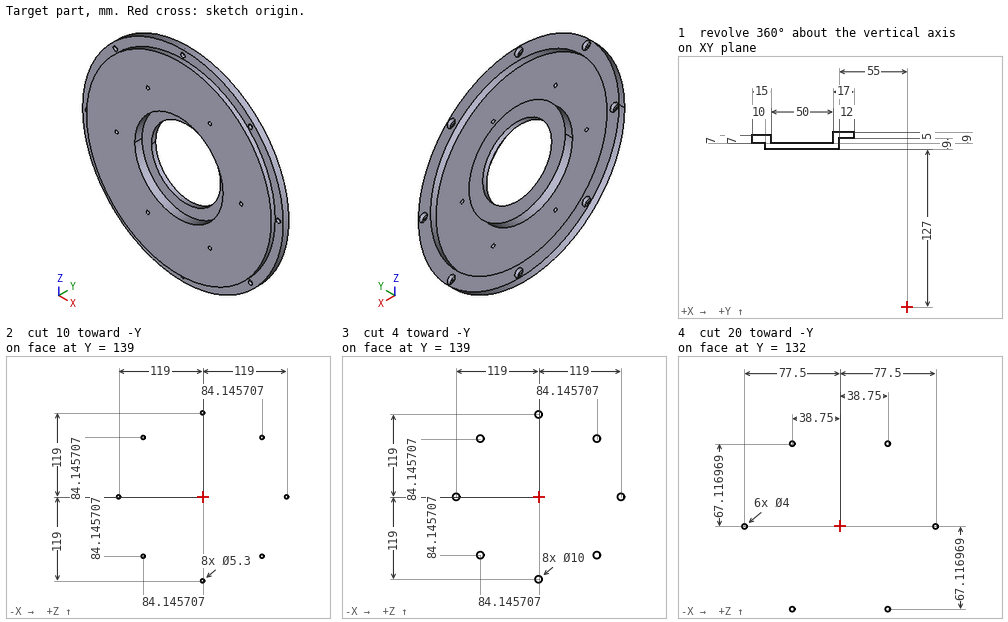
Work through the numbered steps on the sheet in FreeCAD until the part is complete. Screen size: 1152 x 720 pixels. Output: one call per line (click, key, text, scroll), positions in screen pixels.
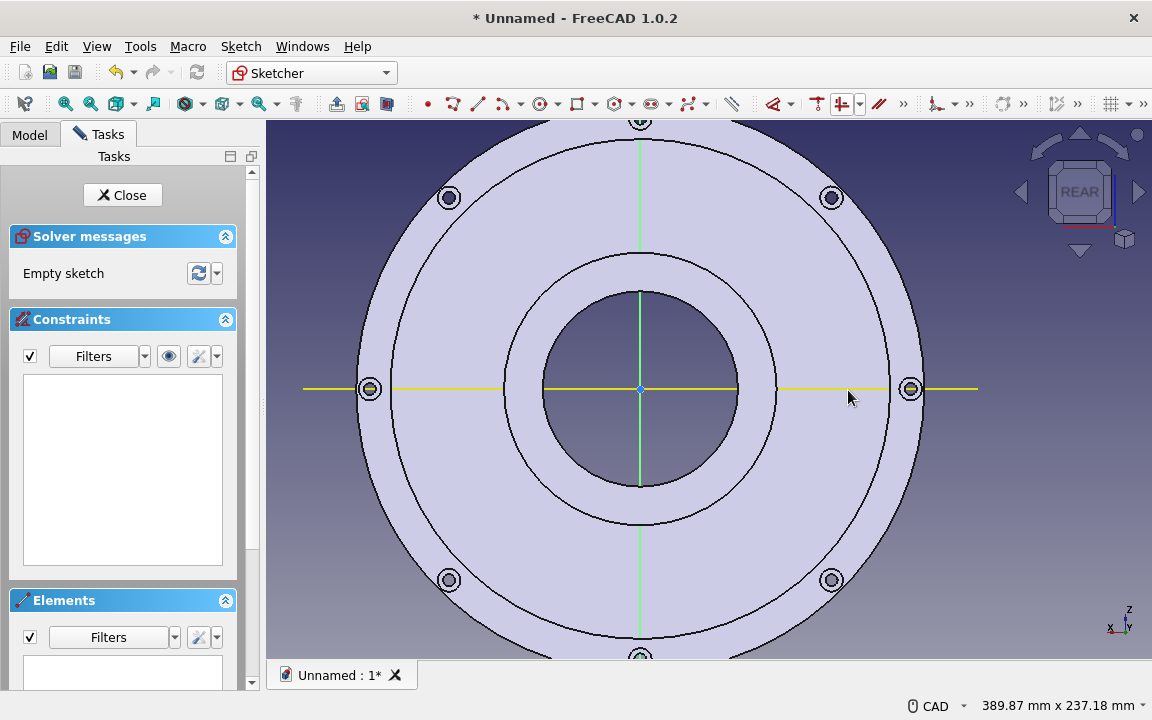
click(540, 104)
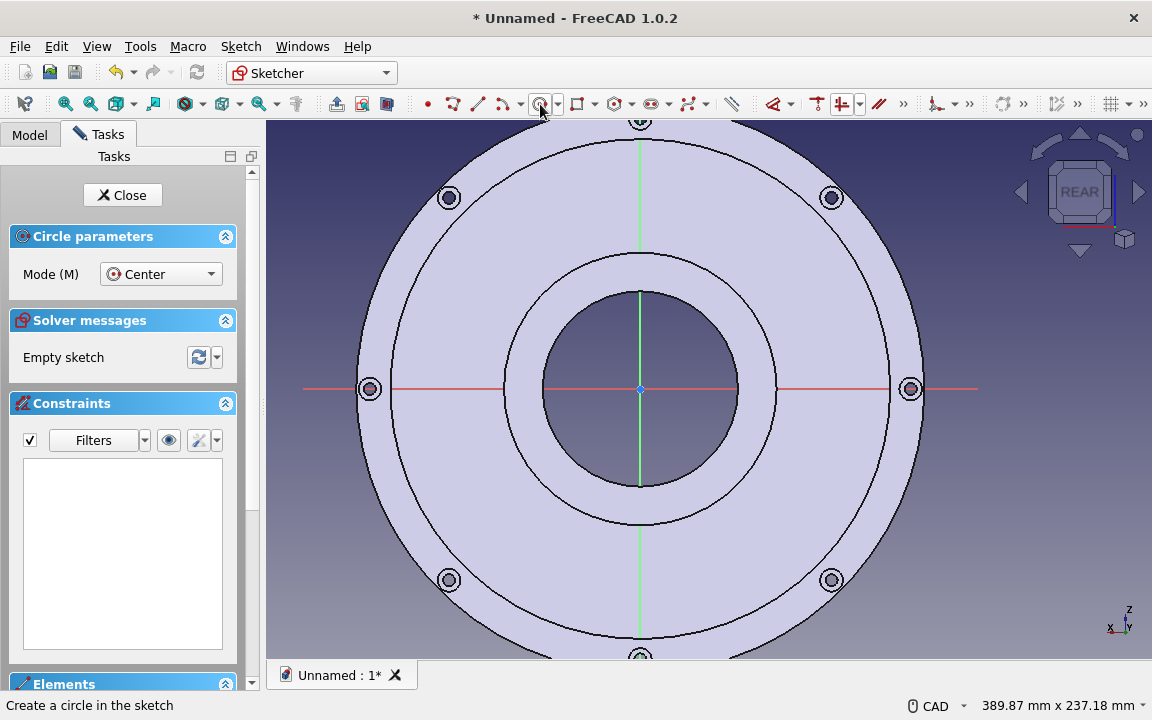
scroll(464, 389, up, 9)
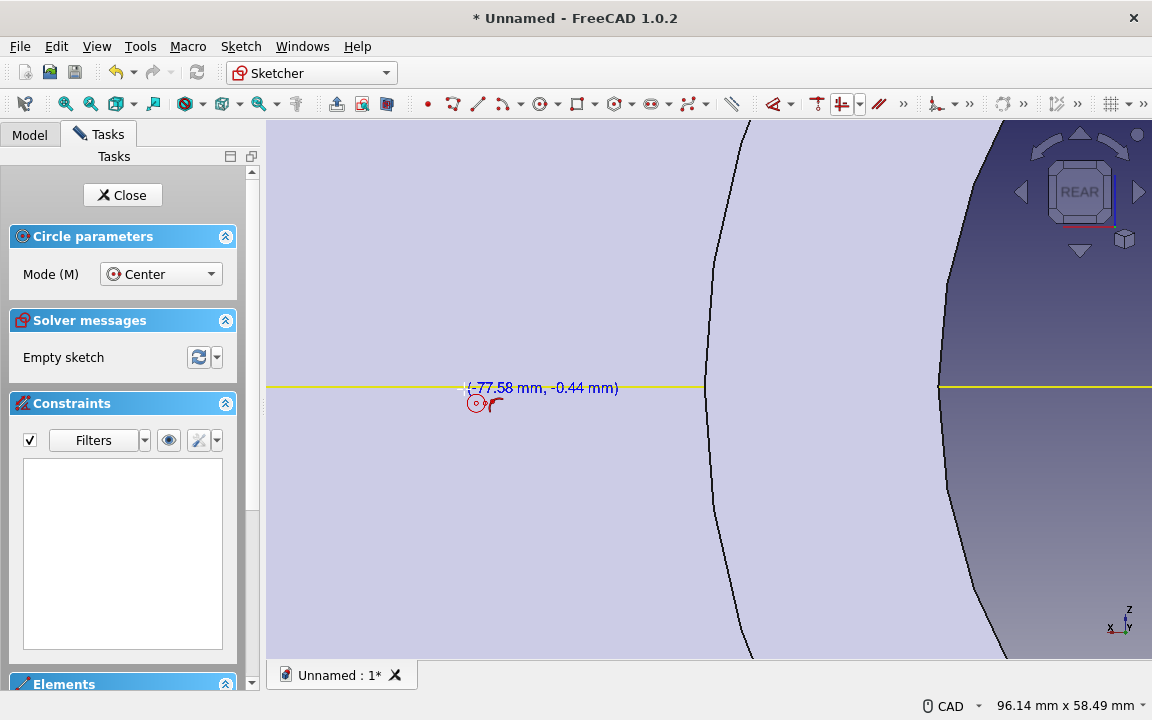
scroll(464, 390, down, 9)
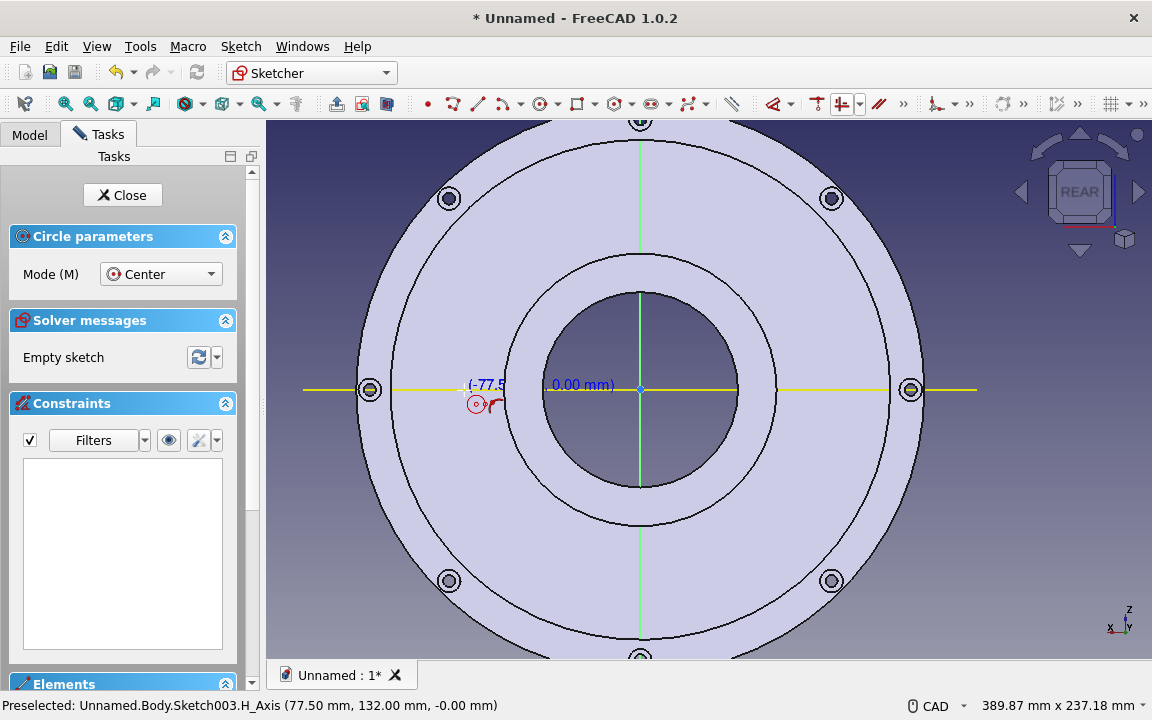
click(464, 390)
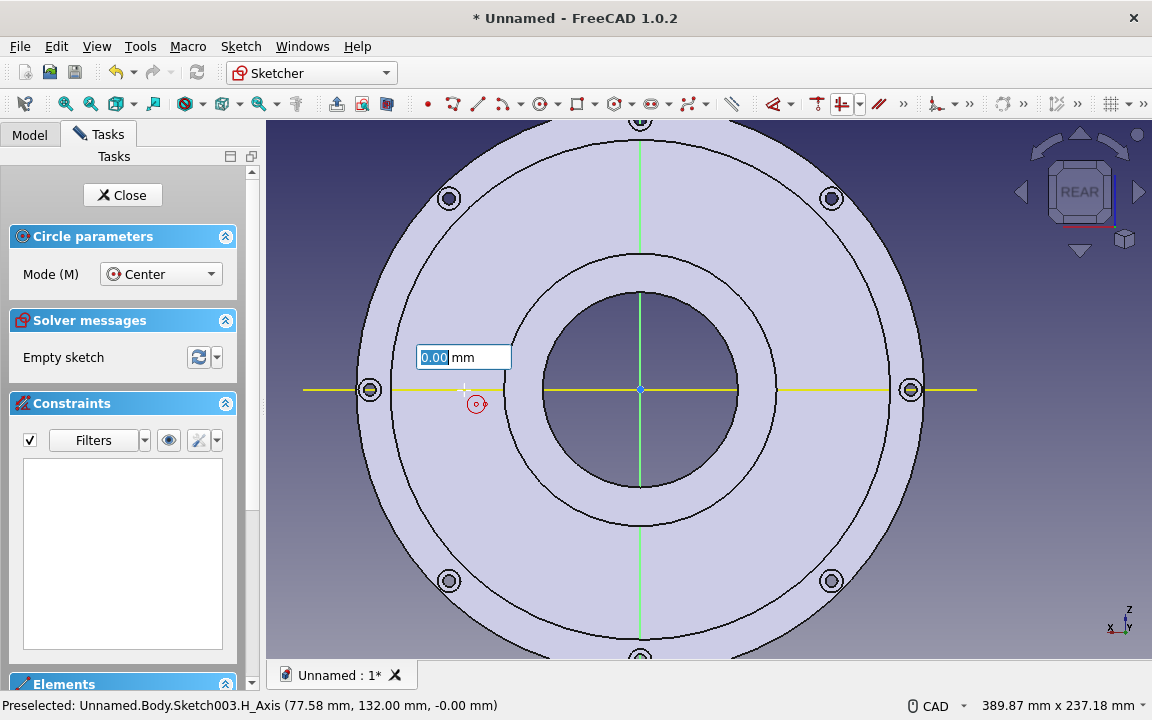
scroll(463, 394, up, 7)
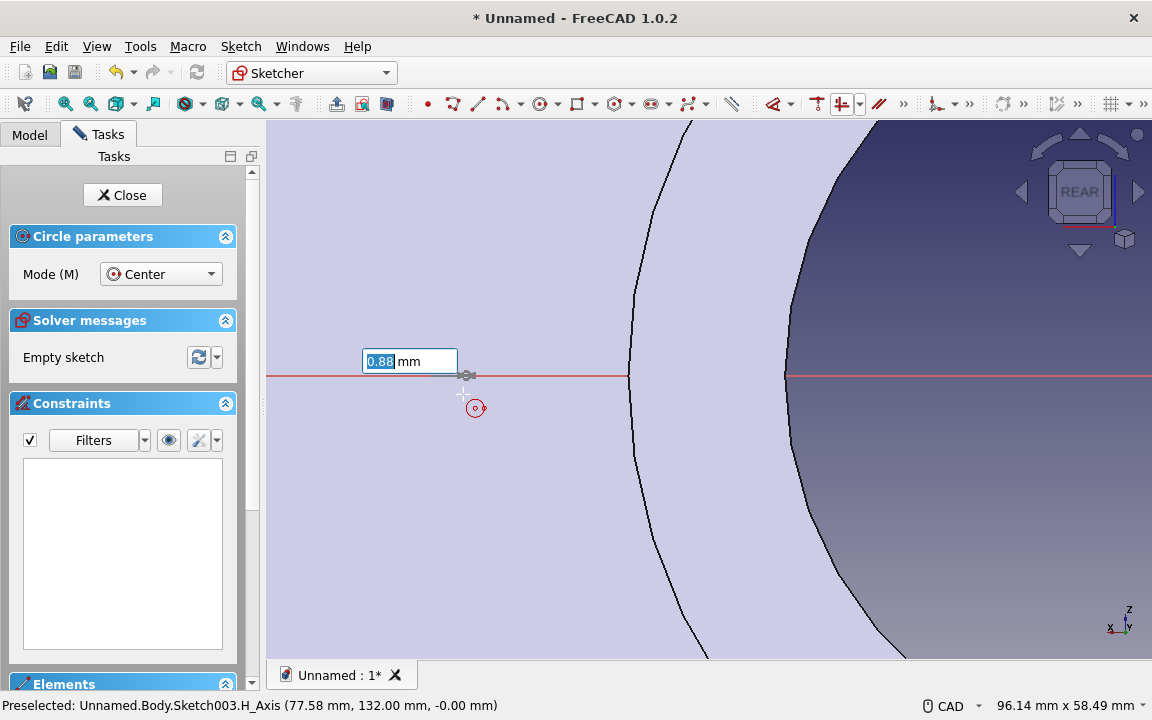
click(461, 393)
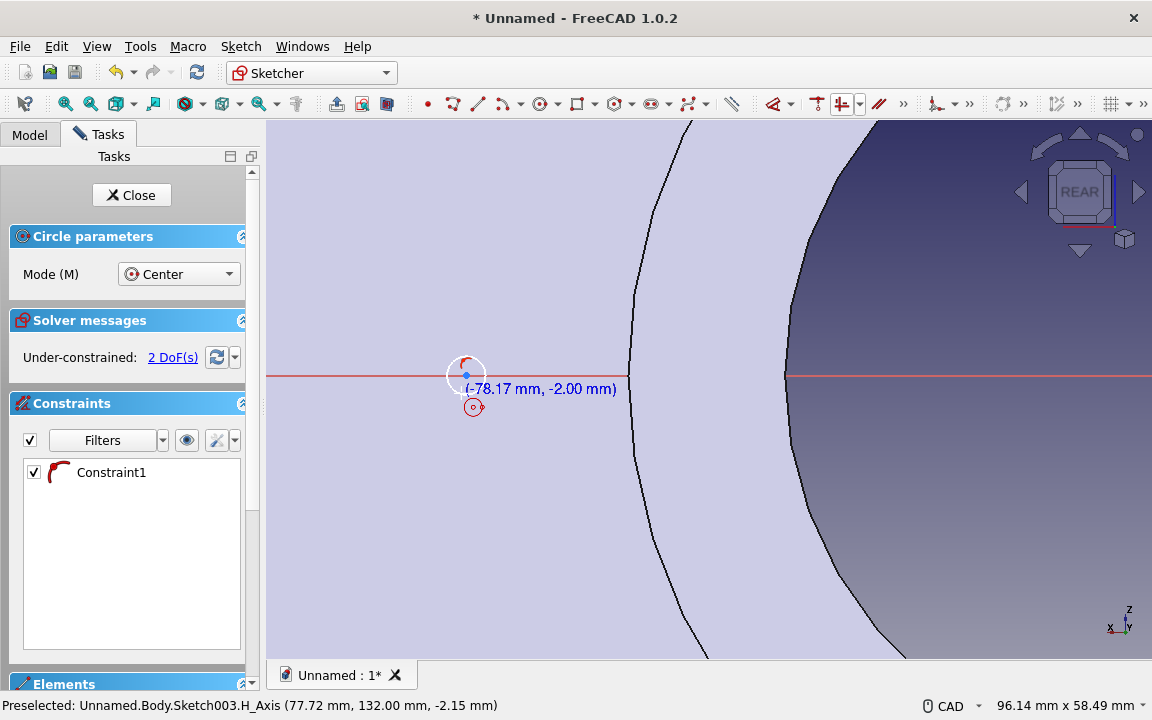
scroll(463, 394, down, 7)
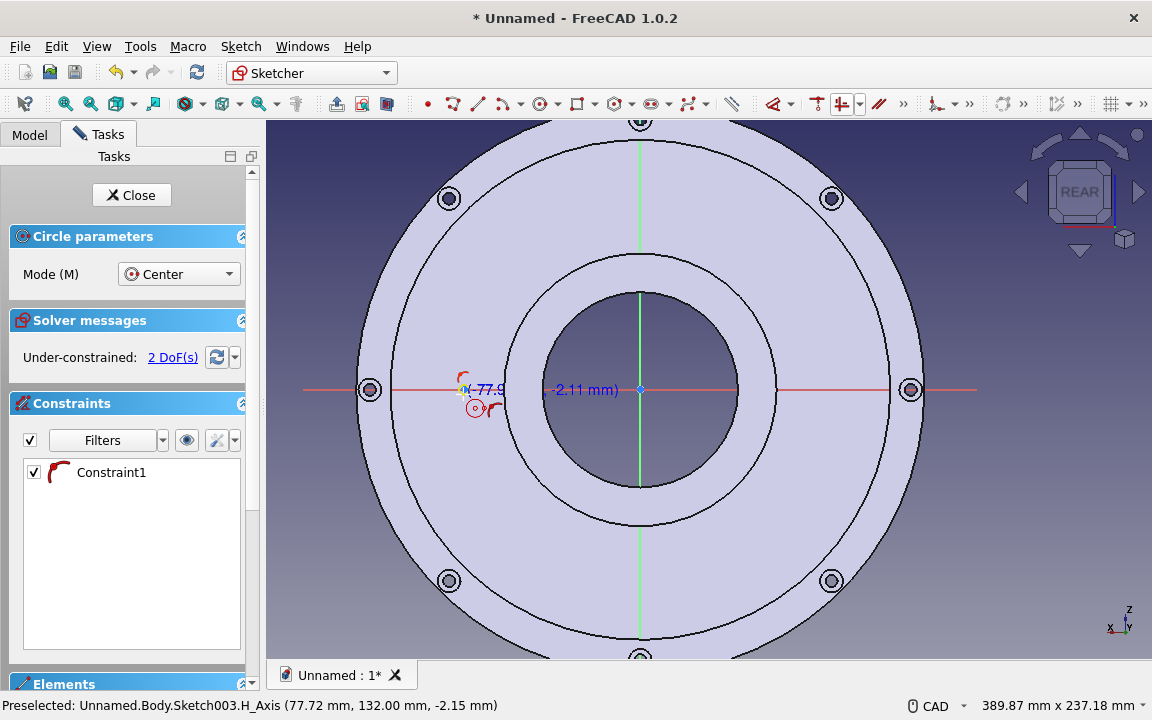
scroll(552, 237, up, 9)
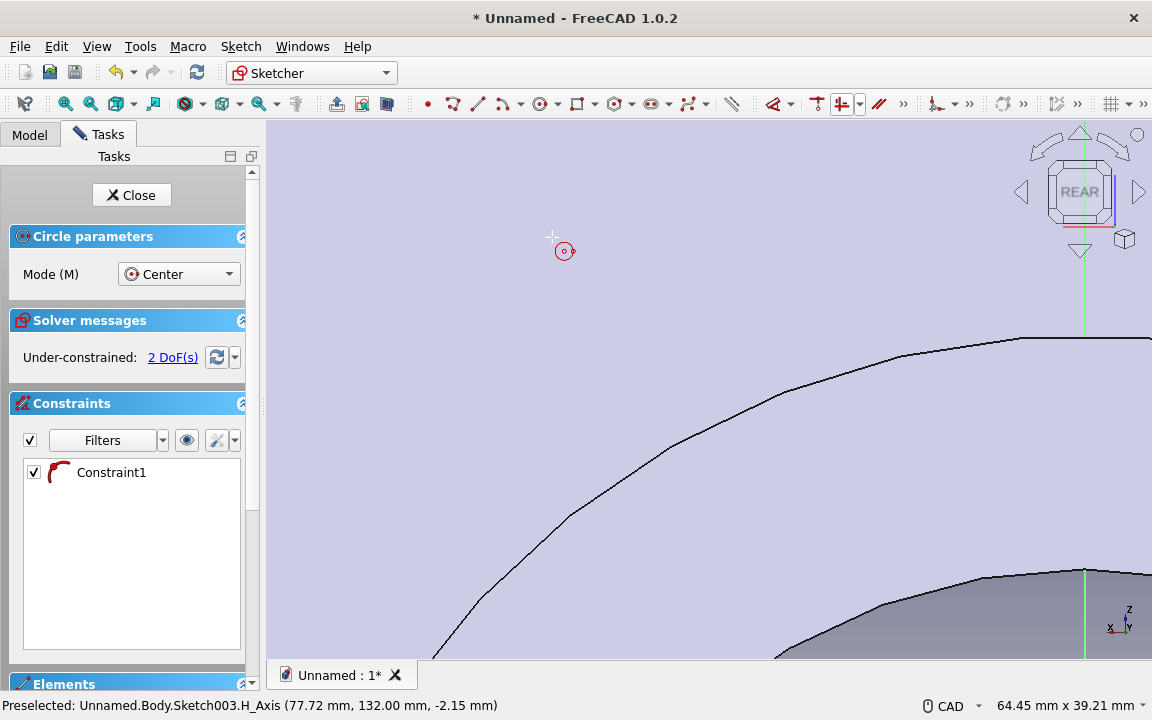
scroll(553, 237, down, 9)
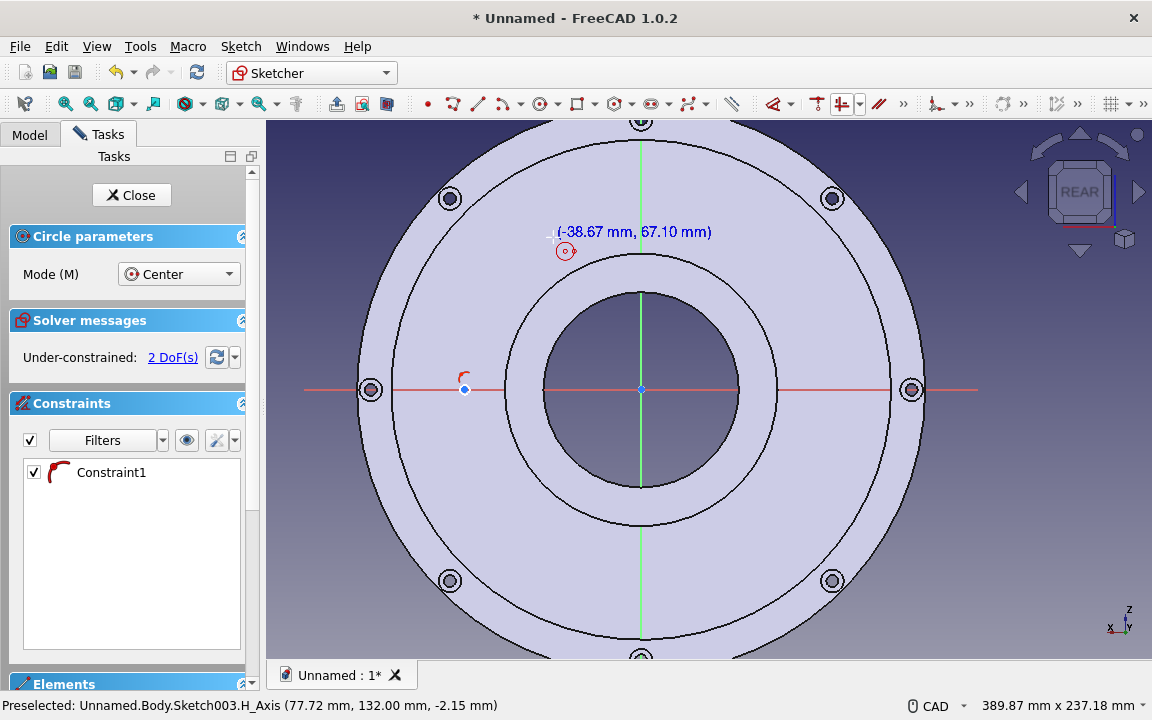
click(553, 237)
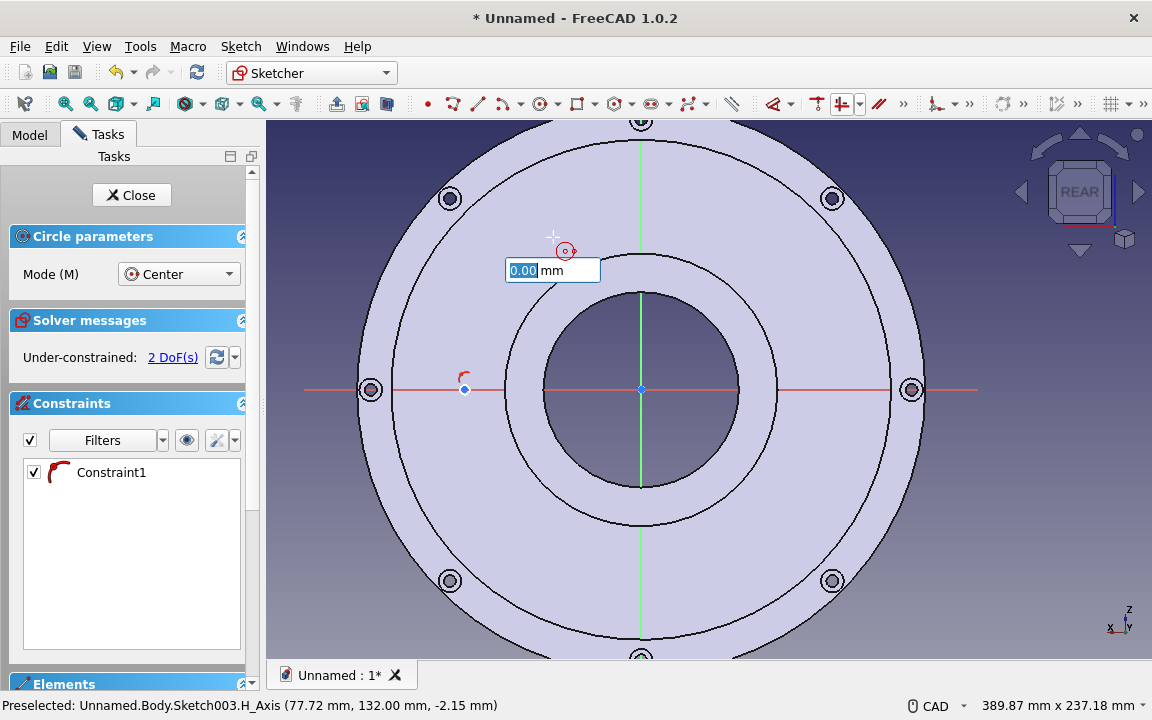
scroll(556, 234, up, 7)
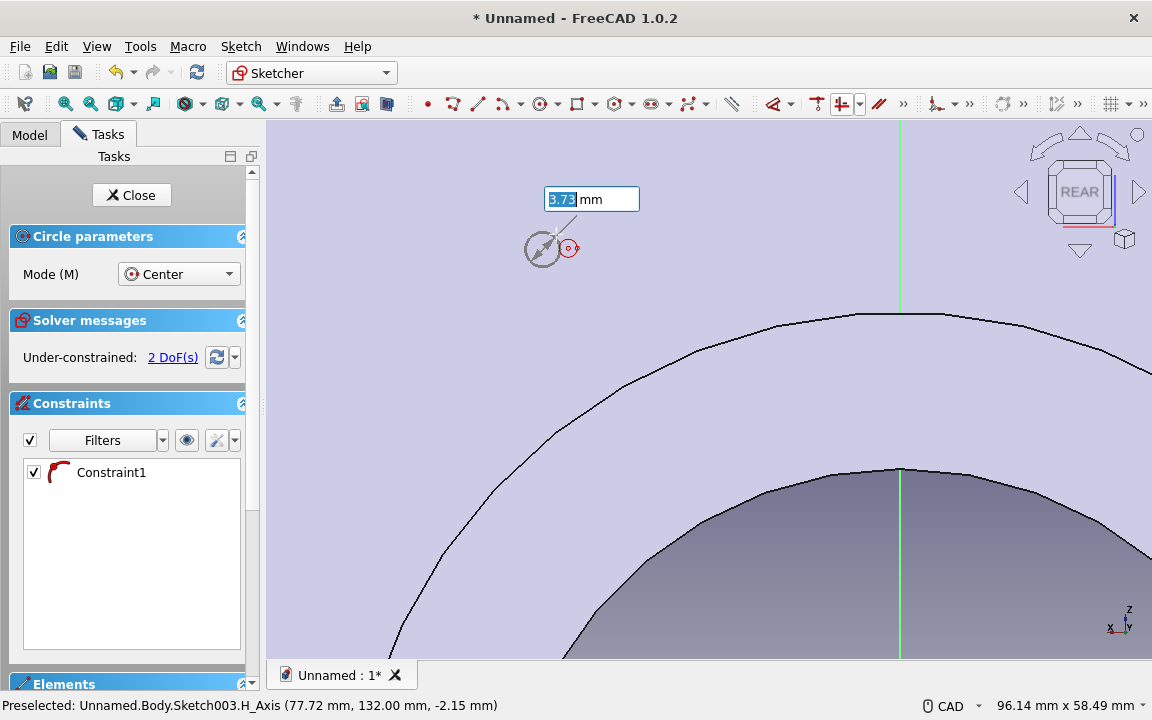
click(556, 234)